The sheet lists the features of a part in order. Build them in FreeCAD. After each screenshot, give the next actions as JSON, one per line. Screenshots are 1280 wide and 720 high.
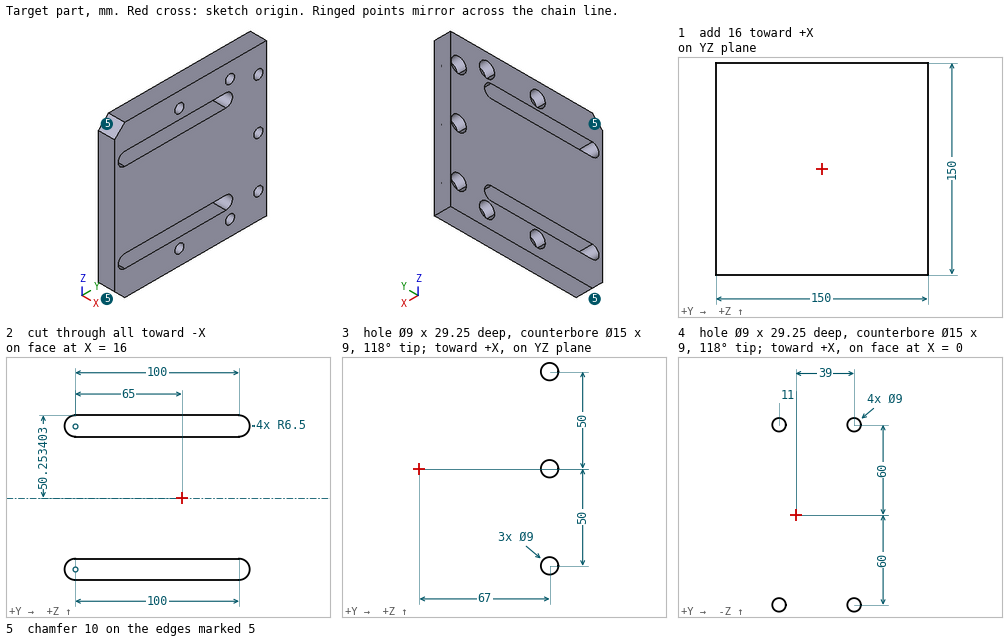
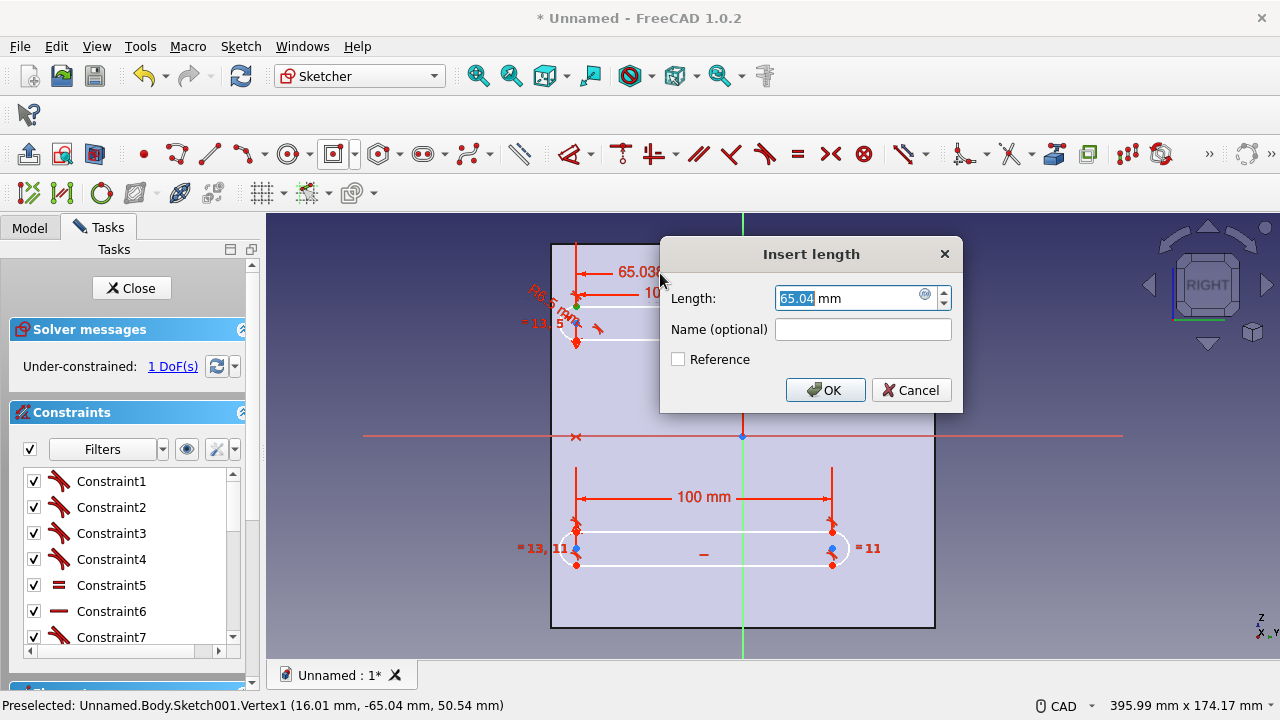
{"action": "type", "text": "65"}
{"action": "key", "text": "Return"}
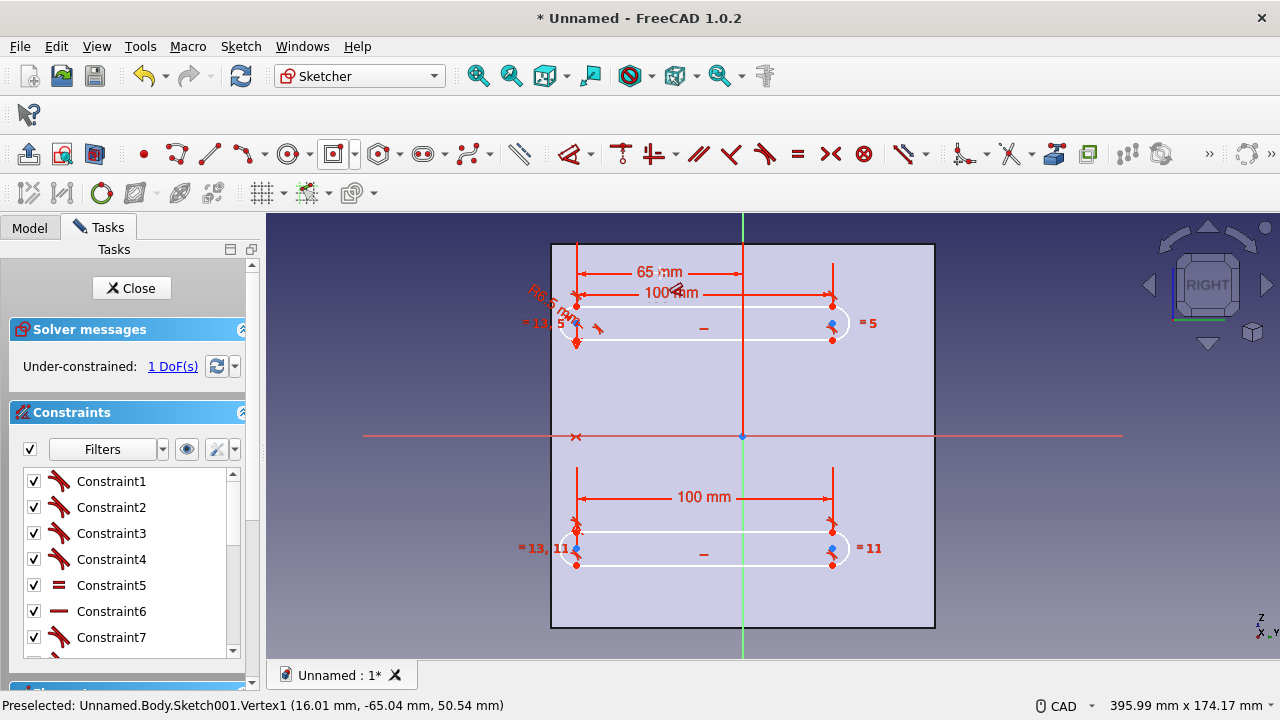
{"action": "left_click", "coordinate": [577, 307]}
{"action": "left_click", "coordinate": [543, 371]}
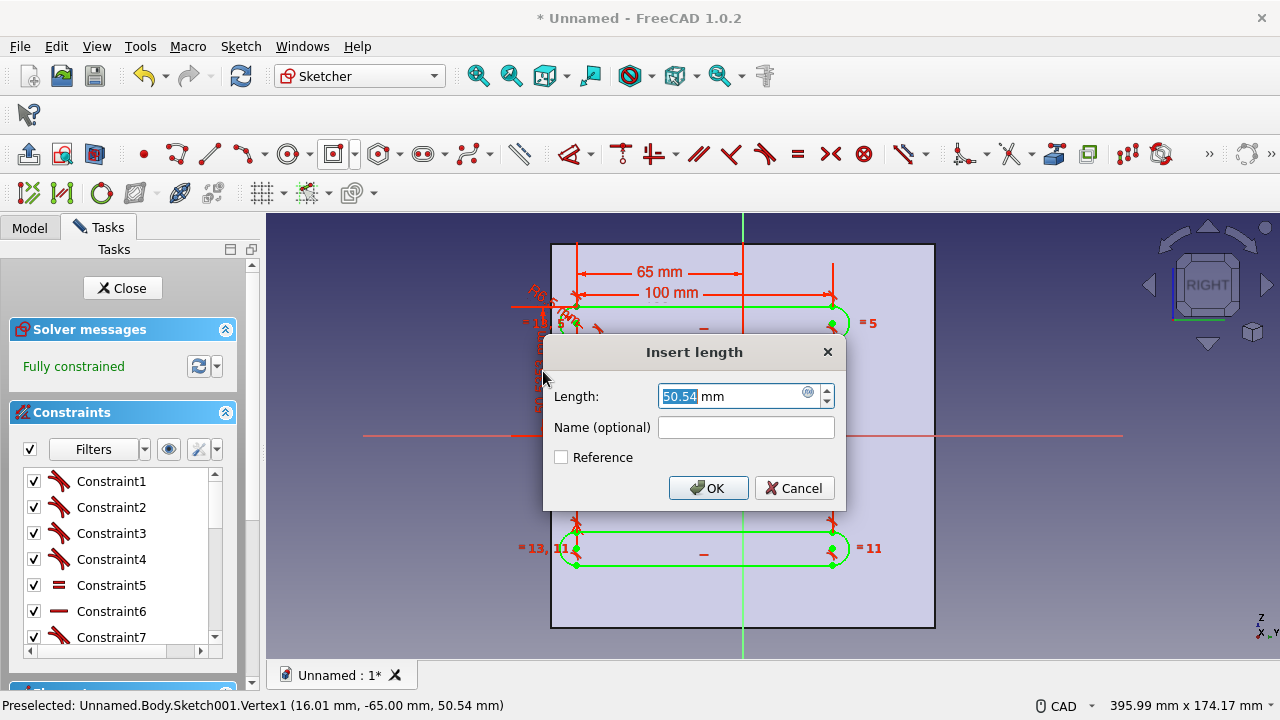
{"action": "type", "text": "50.253403"}
{"action": "key", "text": "Return"}
{"action": "key", "text": "Escape"}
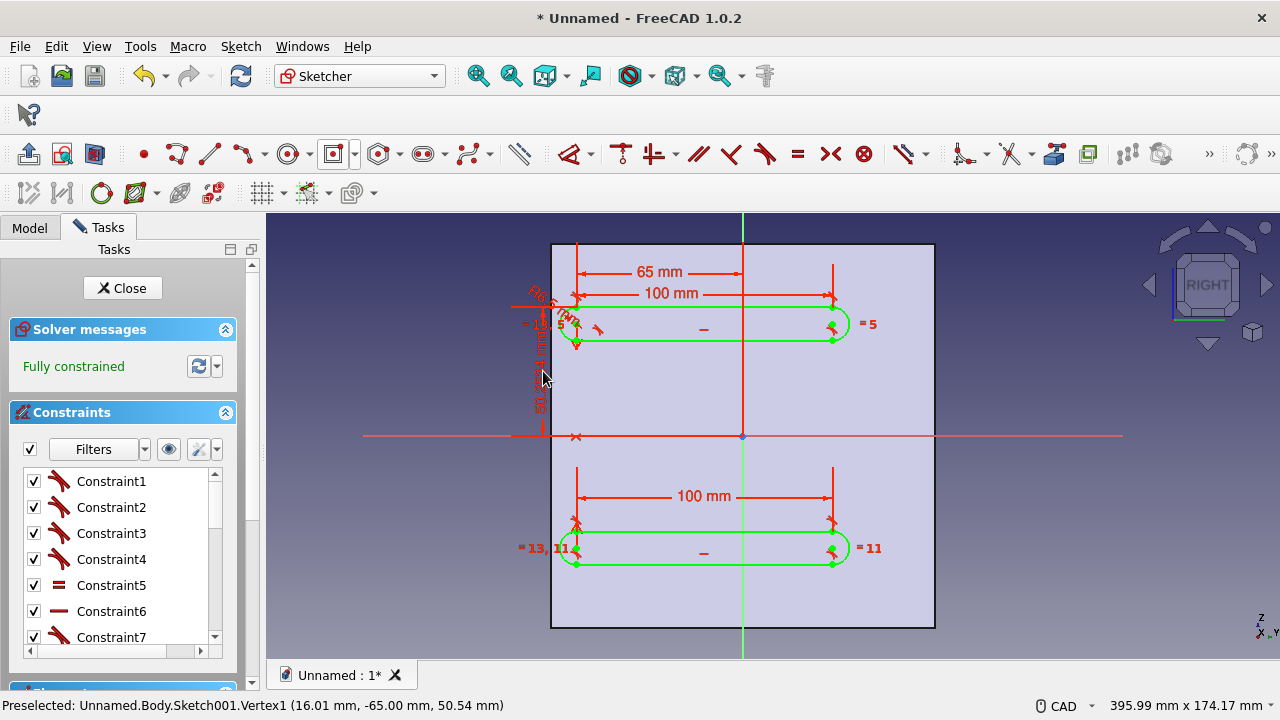
{"action": "left_click", "coordinate": [123, 288]}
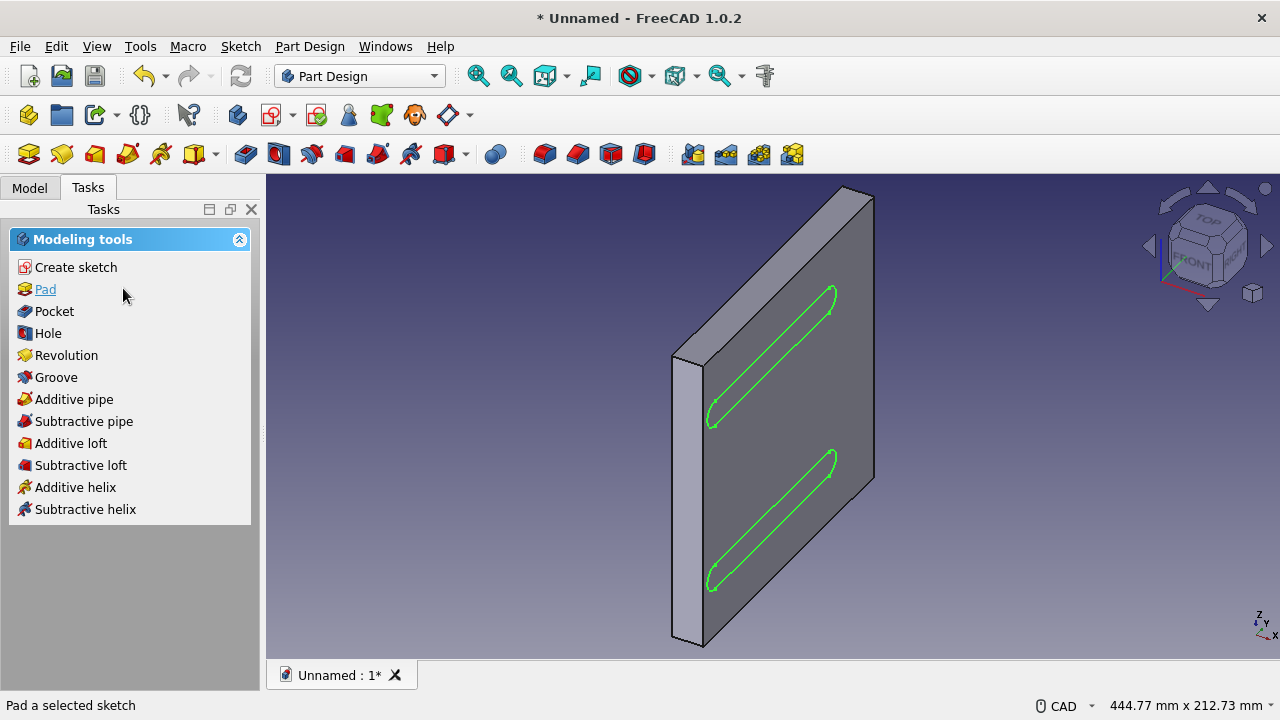
{"action": "left_click", "coordinate": [246, 154]}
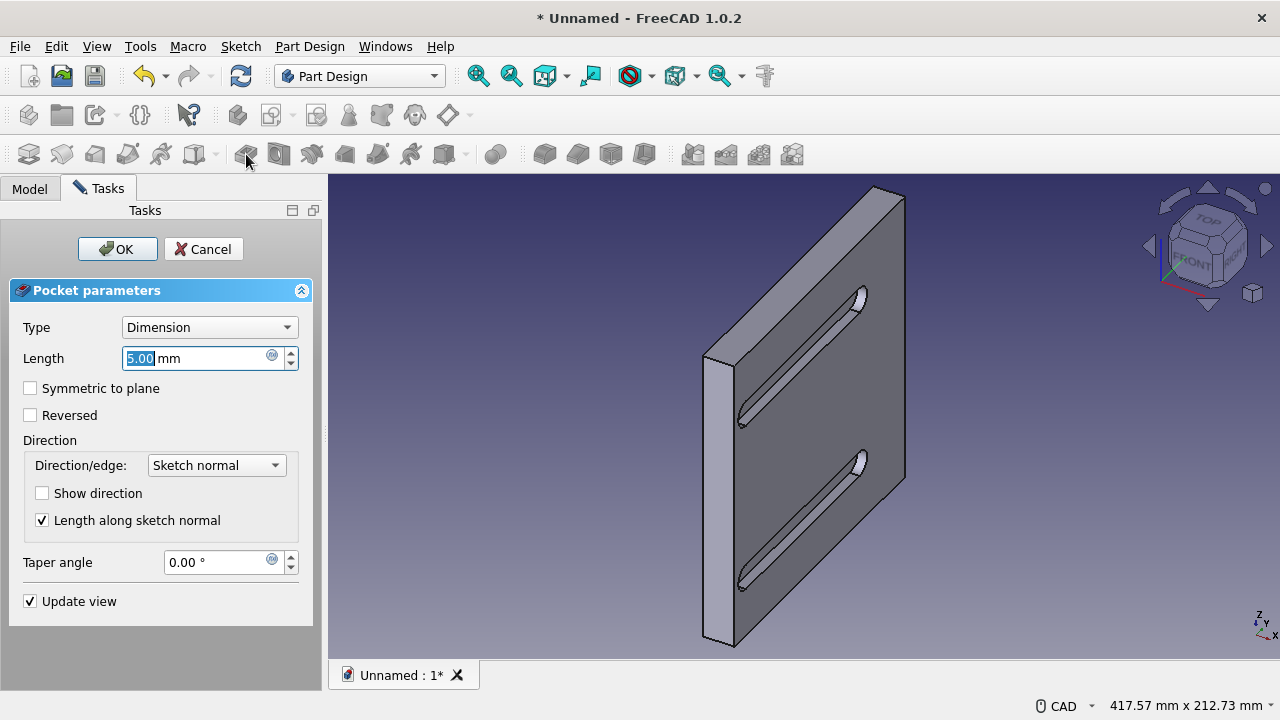
{"action": "left_click", "coordinate": [210, 328]}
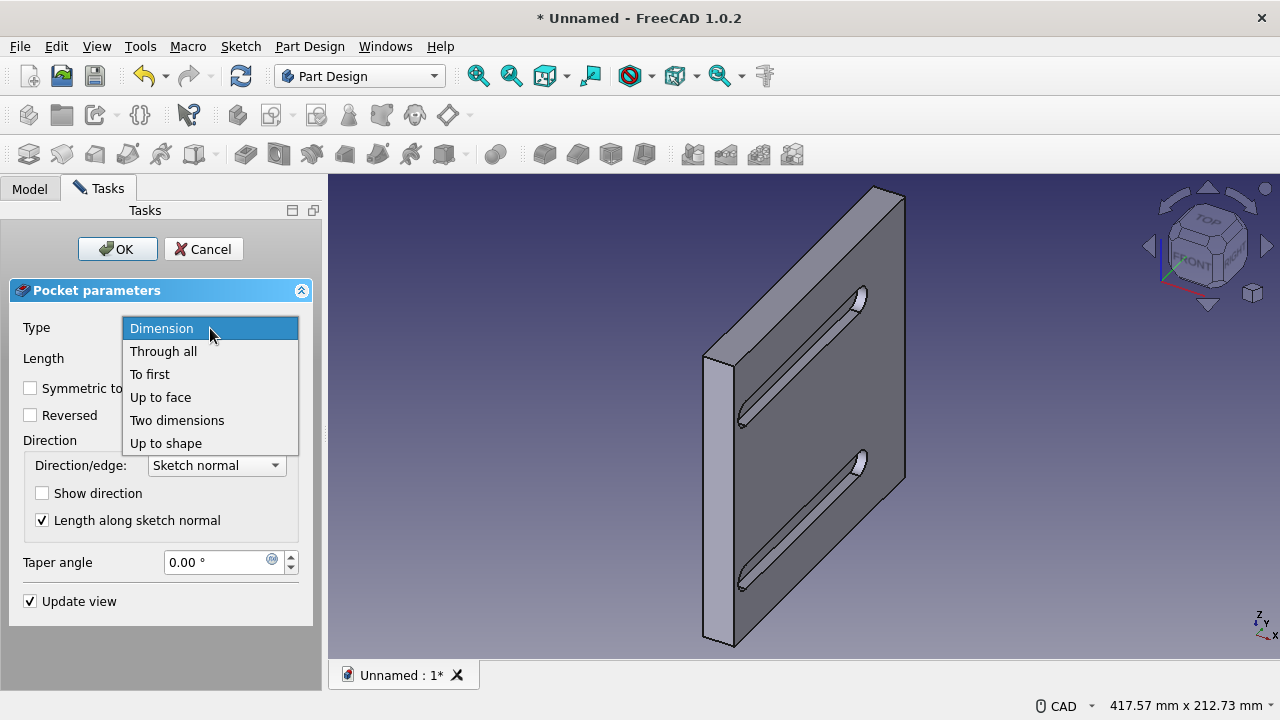
{"action": "left_click", "coordinate": [208, 352]}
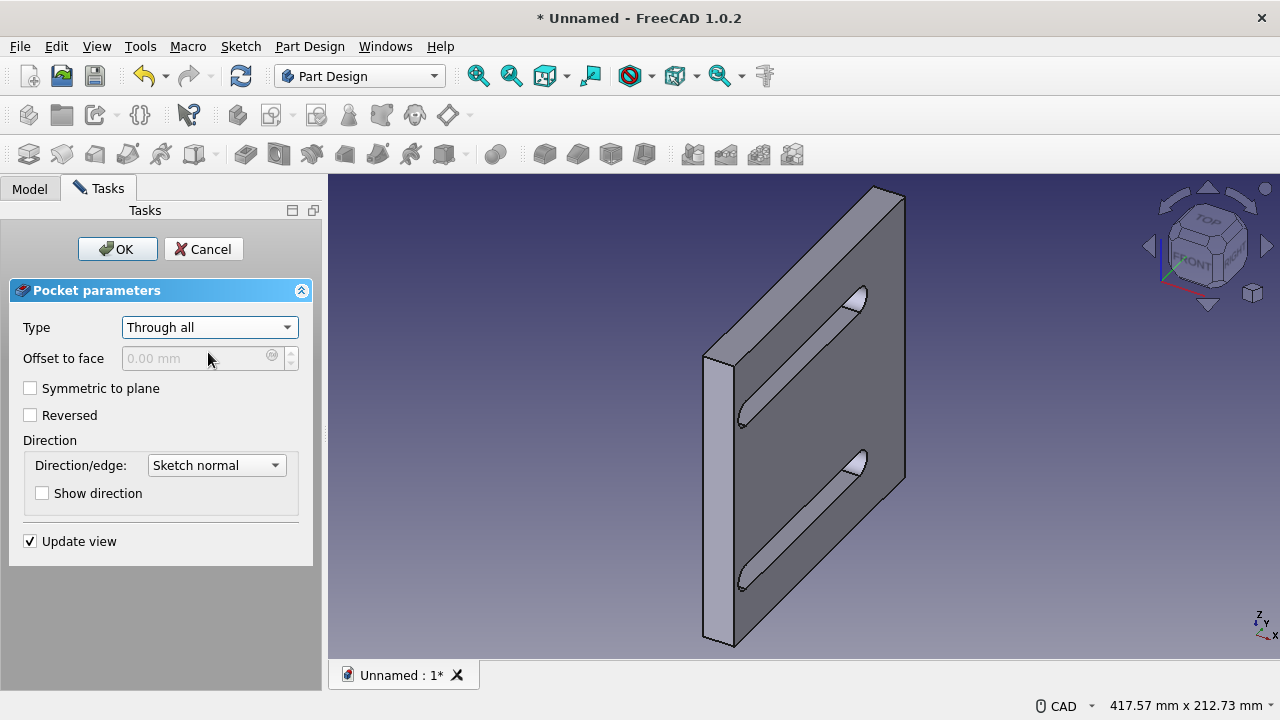
{"action": "left_click", "coordinate": [118, 249]}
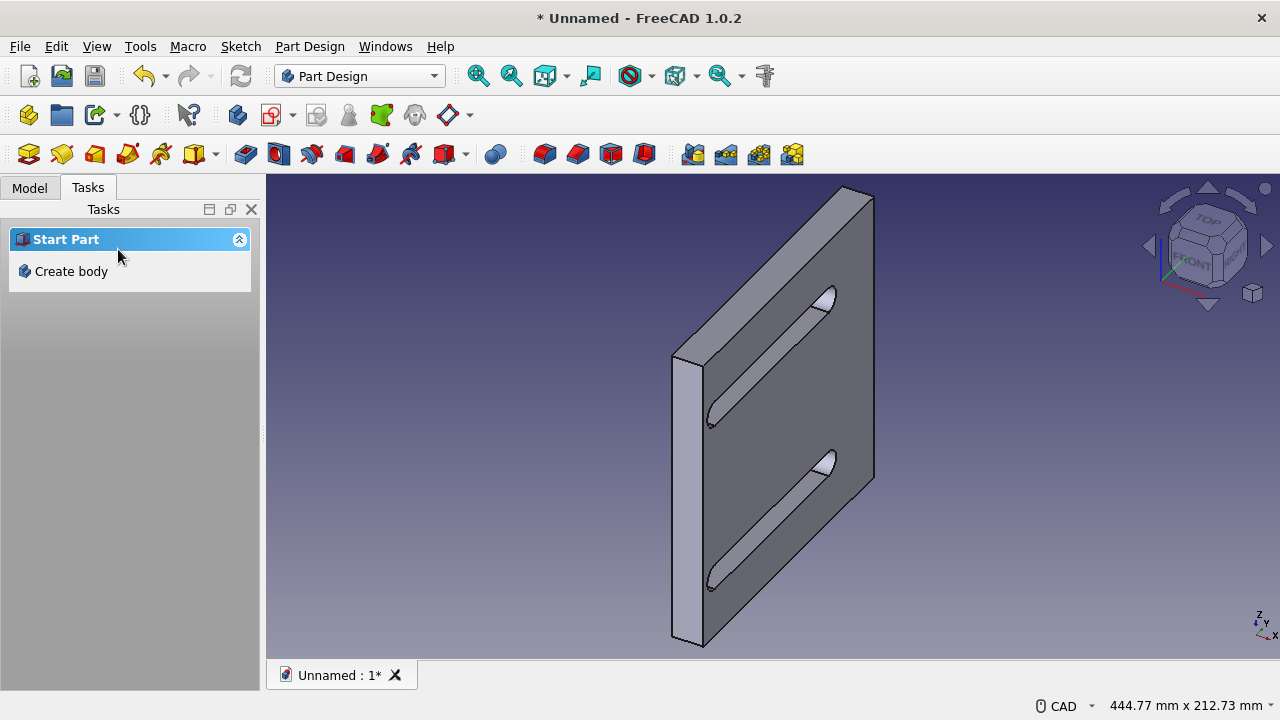
{"action": "left_click", "coordinate": [270, 116]}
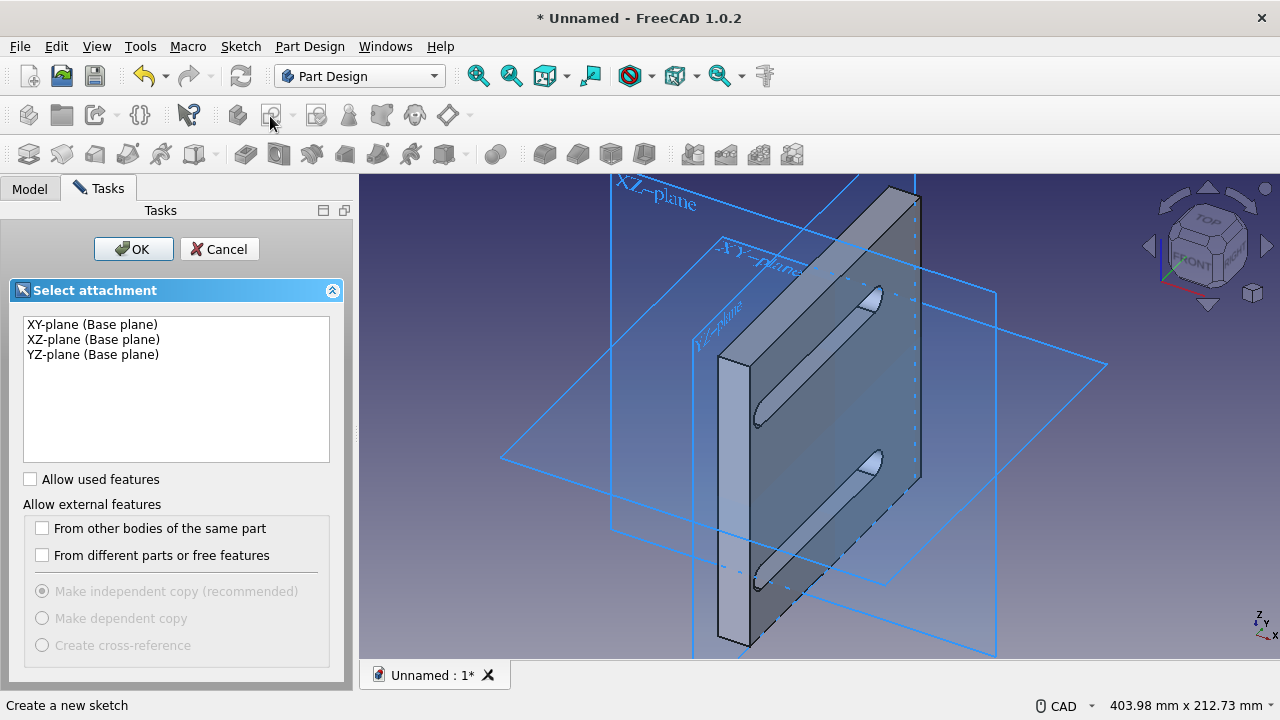
{"action": "left_click", "coordinate": [84, 354]}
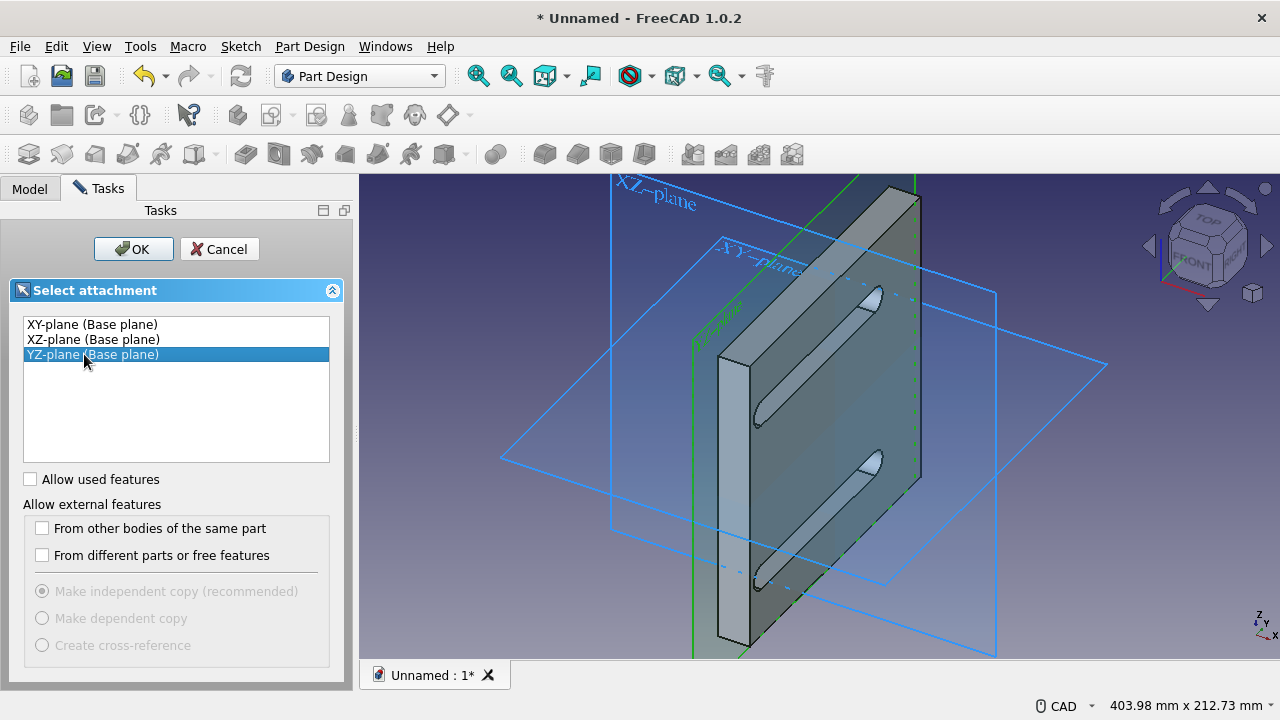
{"action": "left_click", "coordinate": [134, 249]}